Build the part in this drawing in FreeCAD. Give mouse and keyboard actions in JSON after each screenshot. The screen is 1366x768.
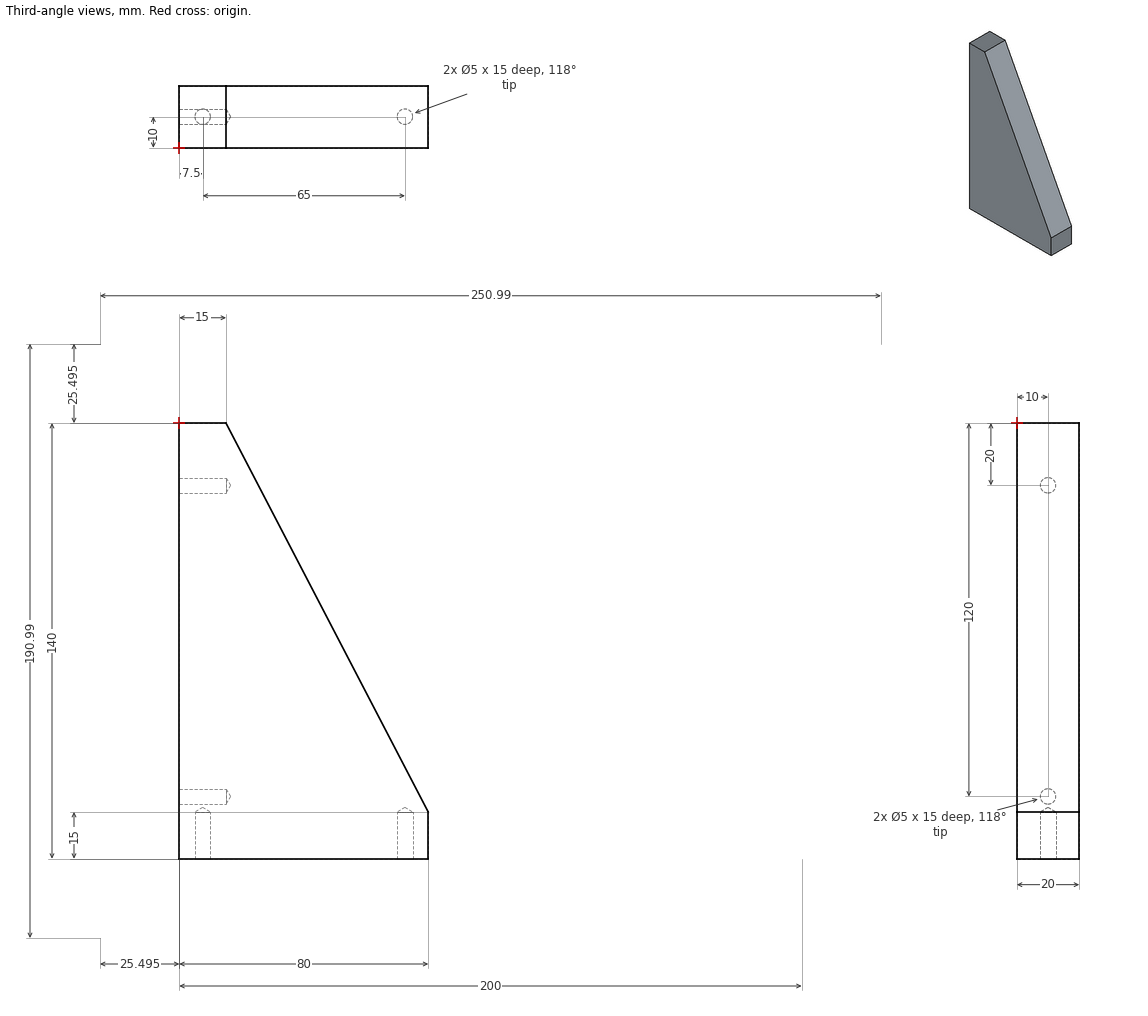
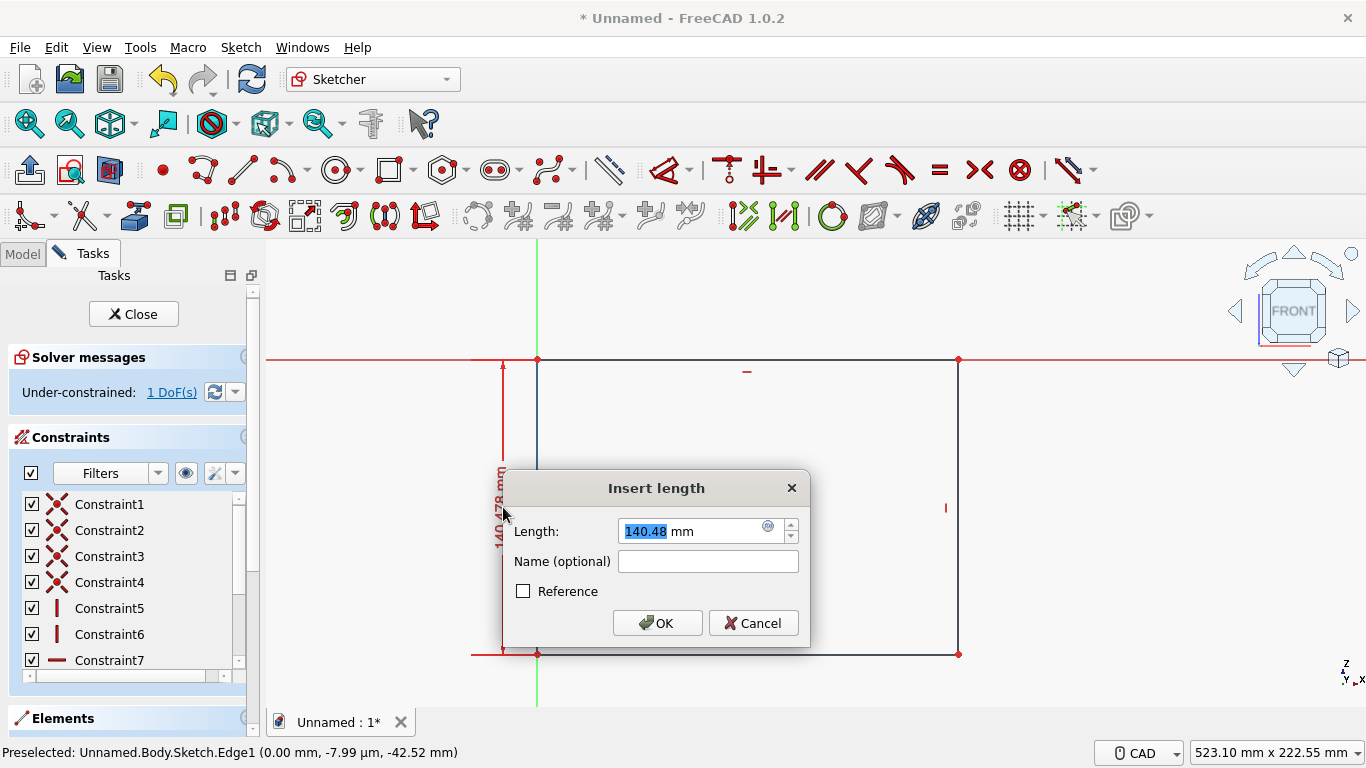
{"action": "type", "text": "140"}
{"action": "key", "text": "Return"}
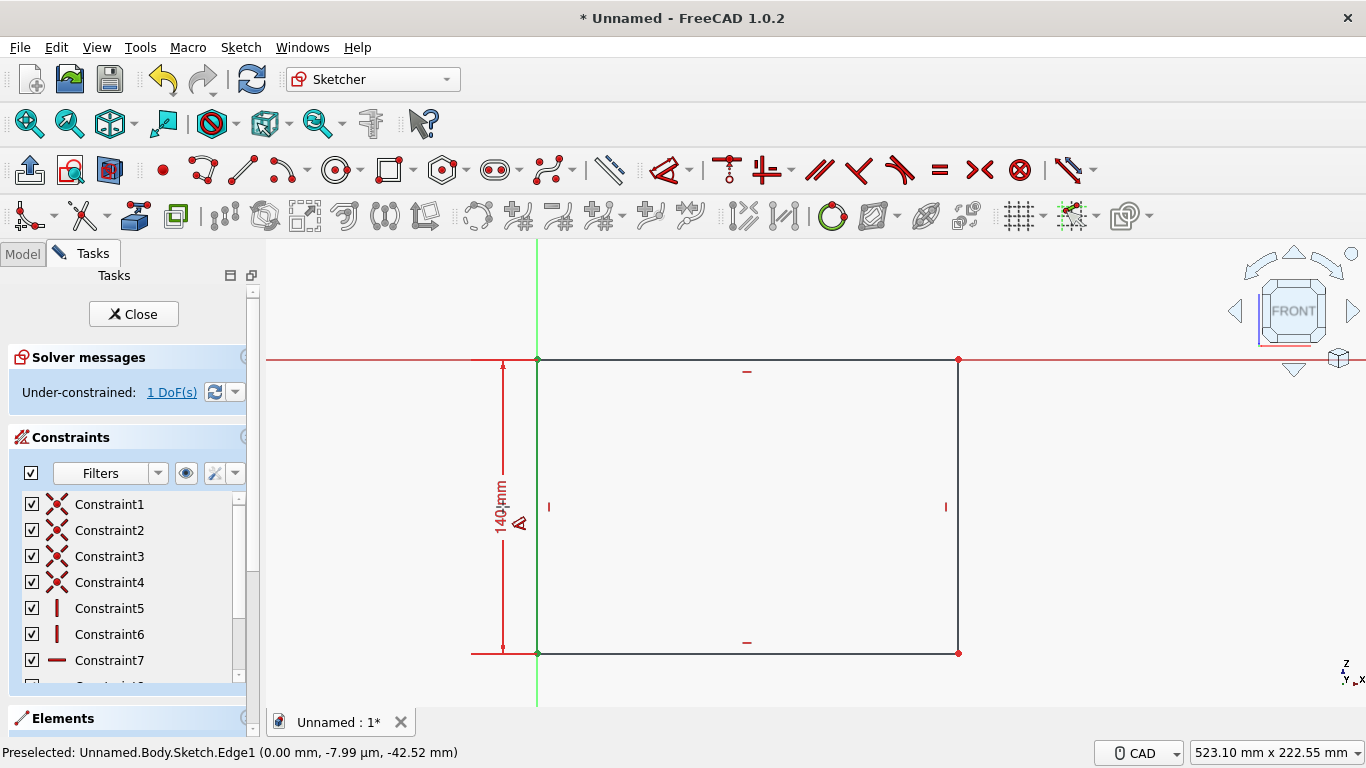
{"action": "left_click", "coordinate": [664, 654]}
{"action": "left_click", "coordinate": [748, 620]}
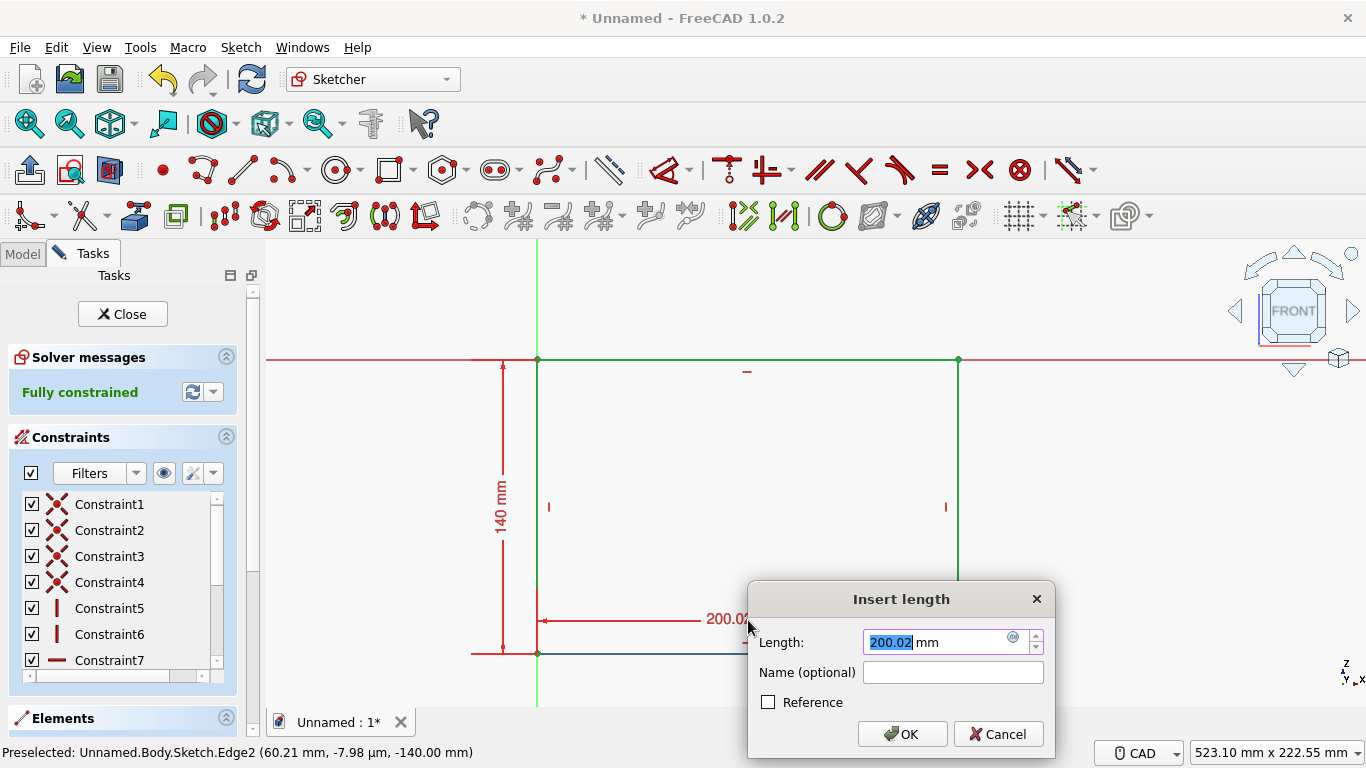
{"action": "type", "text": "200"}
{"action": "key", "text": "Return"}
{"action": "key", "text": "Escape"}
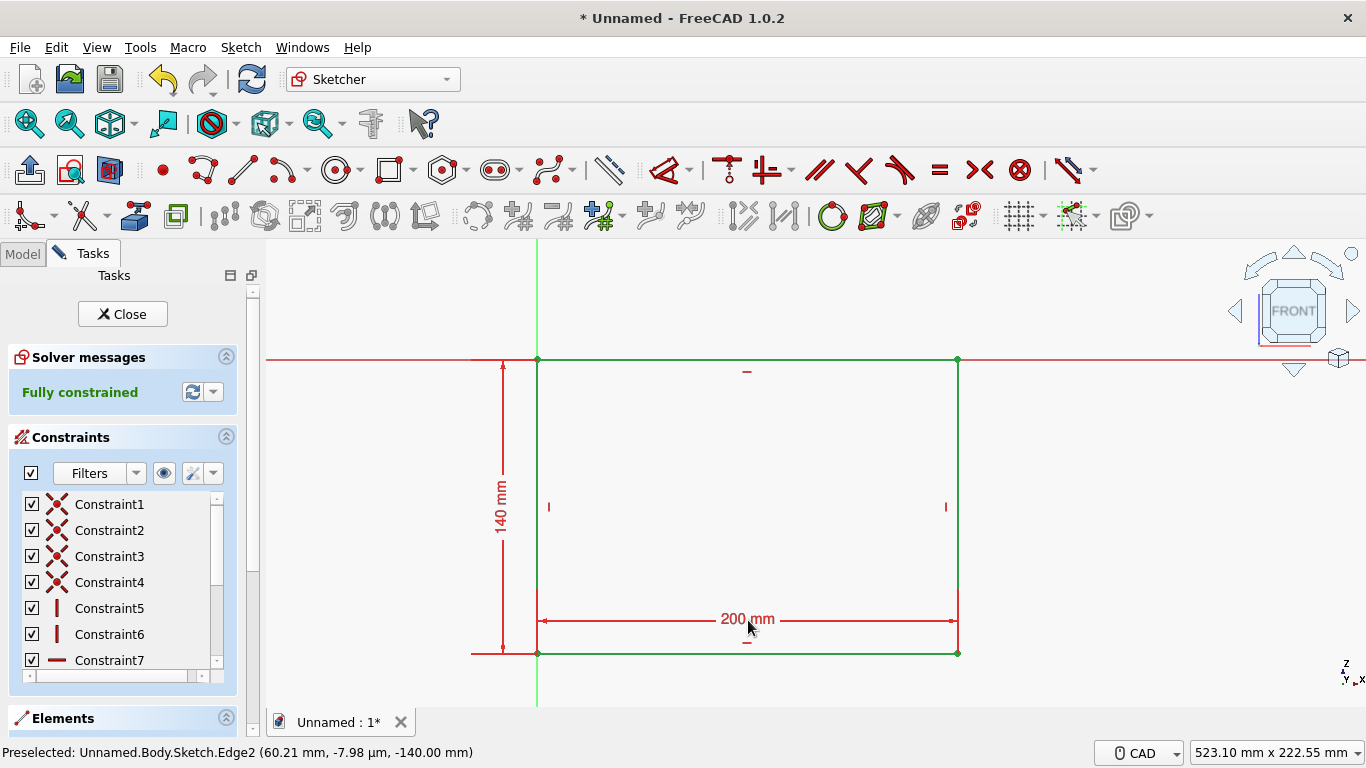
{"action": "left_click", "coordinate": [123, 314]}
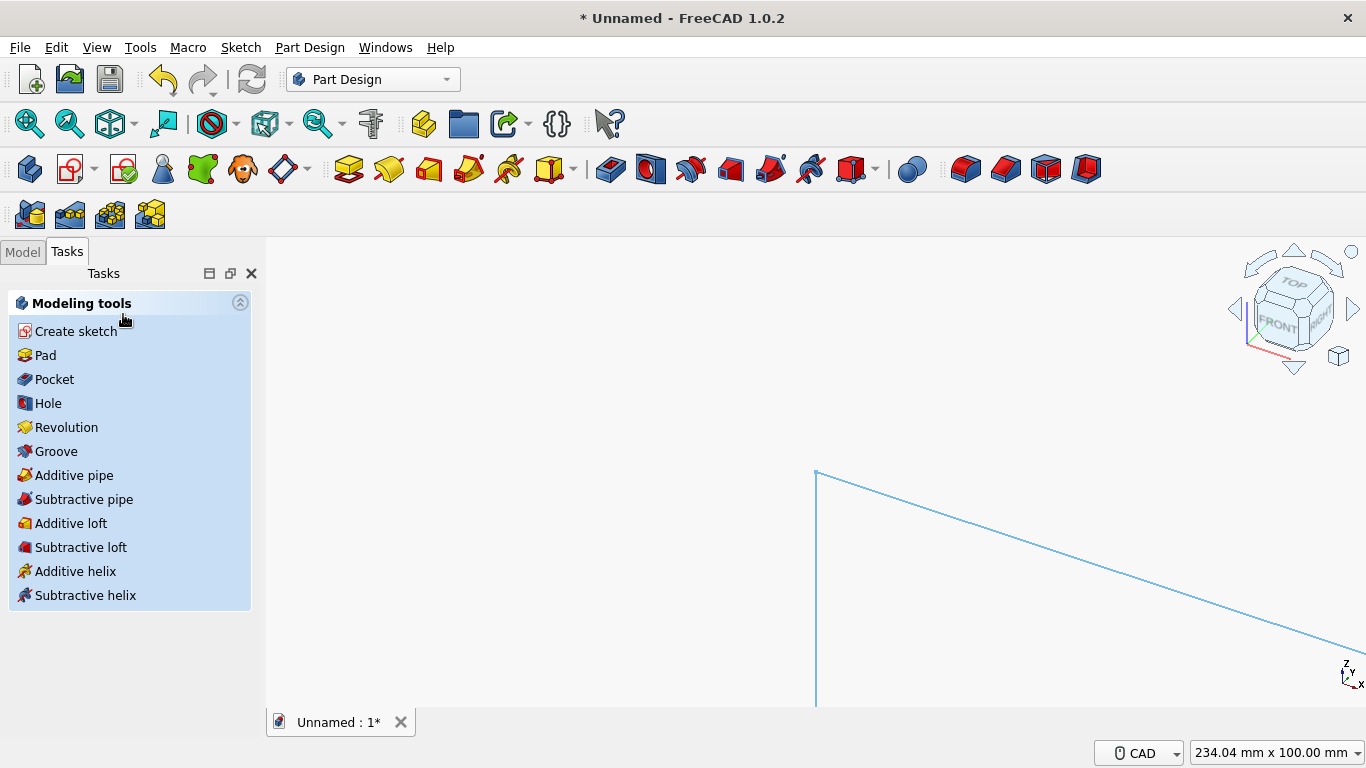
{"action": "left_click", "coordinate": [350, 170]}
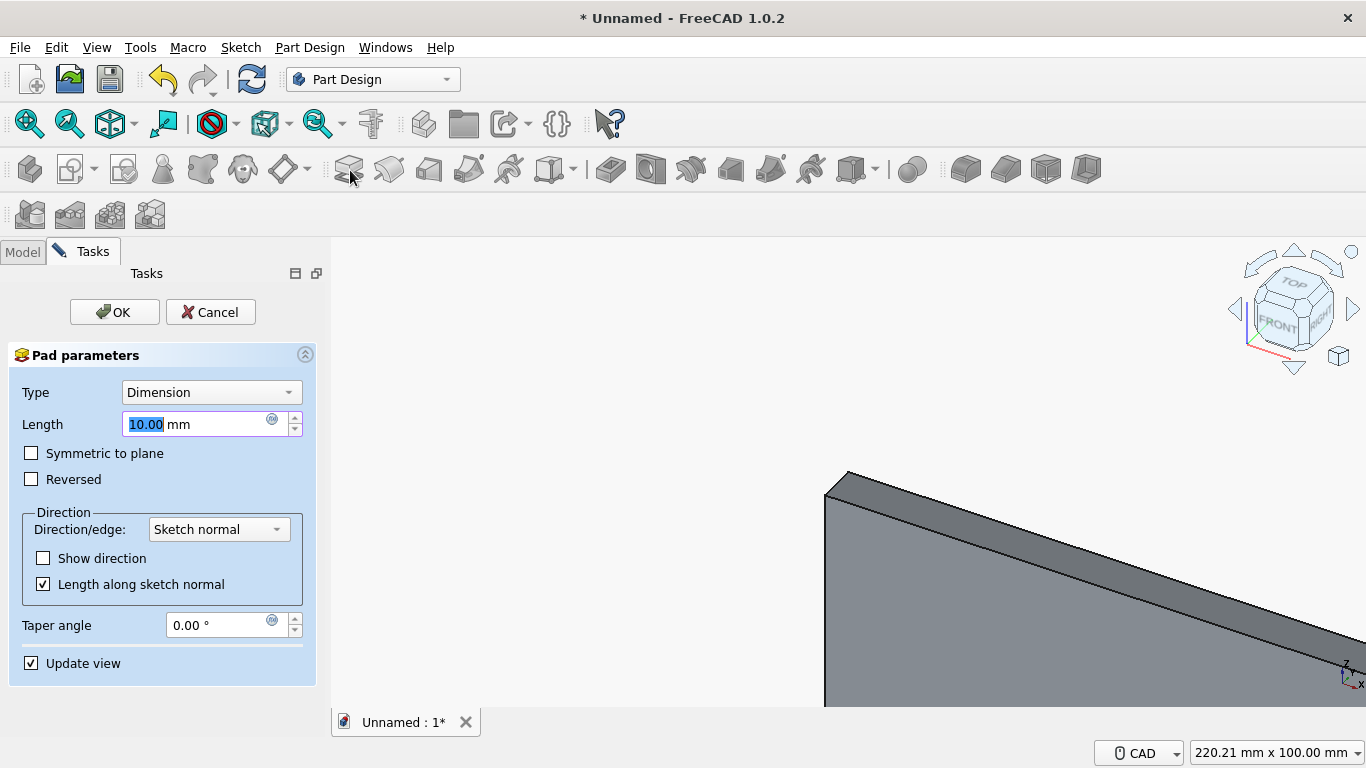
{"action": "type", "text": "20"}
{"action": "key", "text": "Tab"}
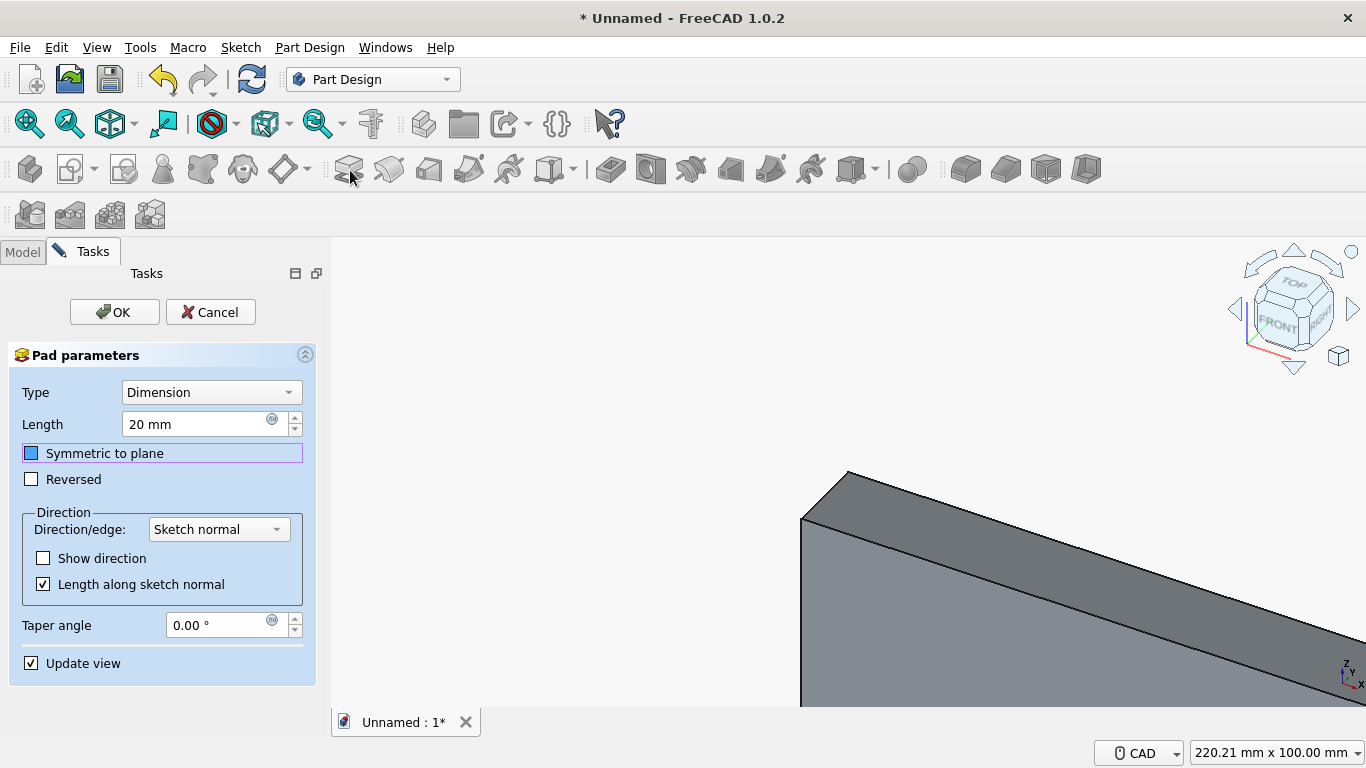
{"action": "left_click", "coordinate": [30, 479]}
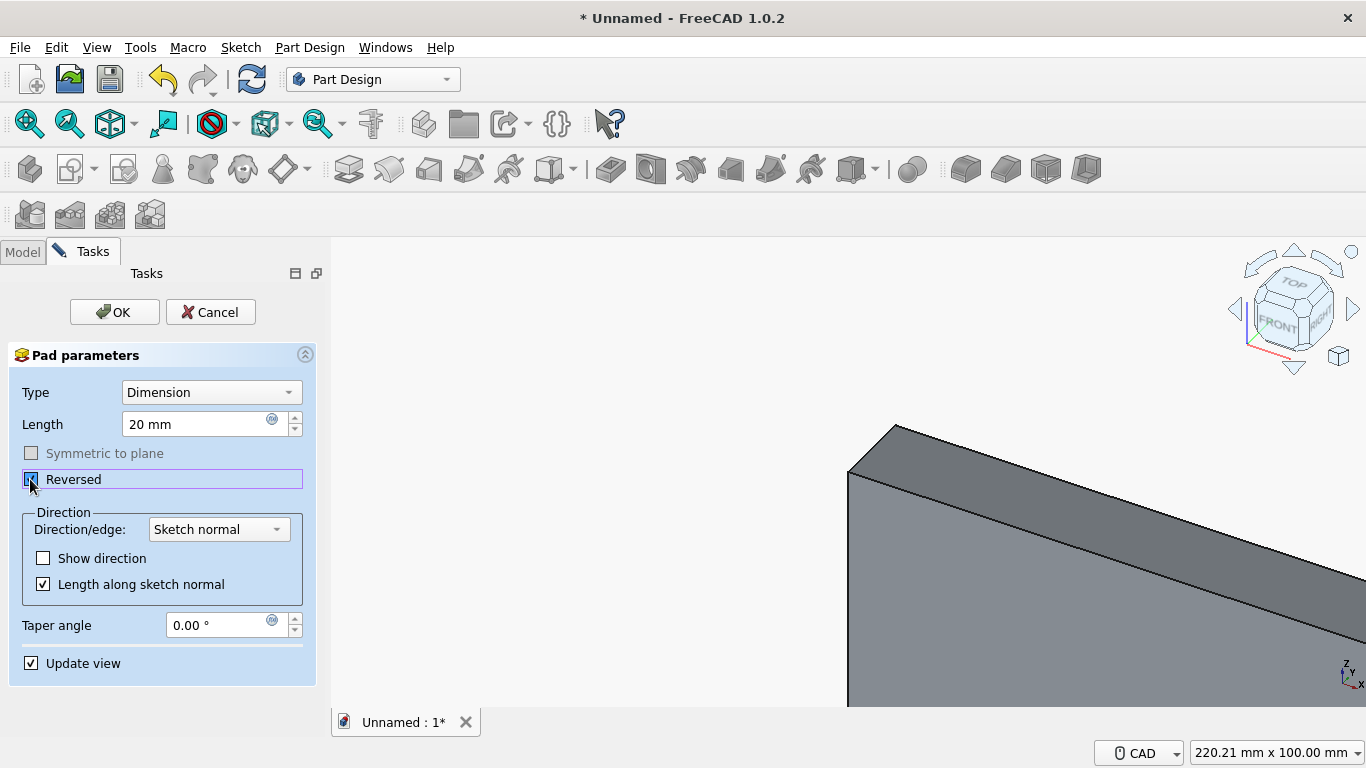
{"action": "left_click", "coordinate": [115, 312]}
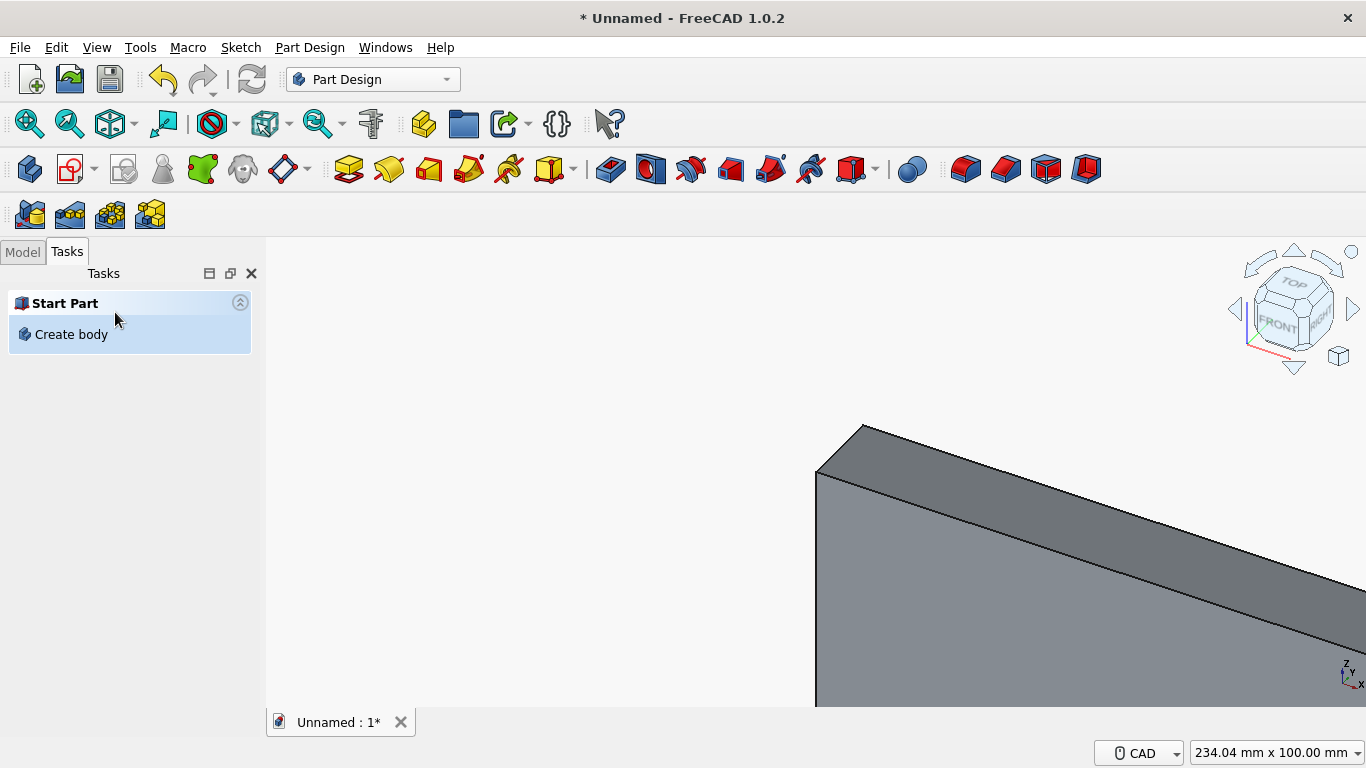
{"action": "key", "text": "v f"}